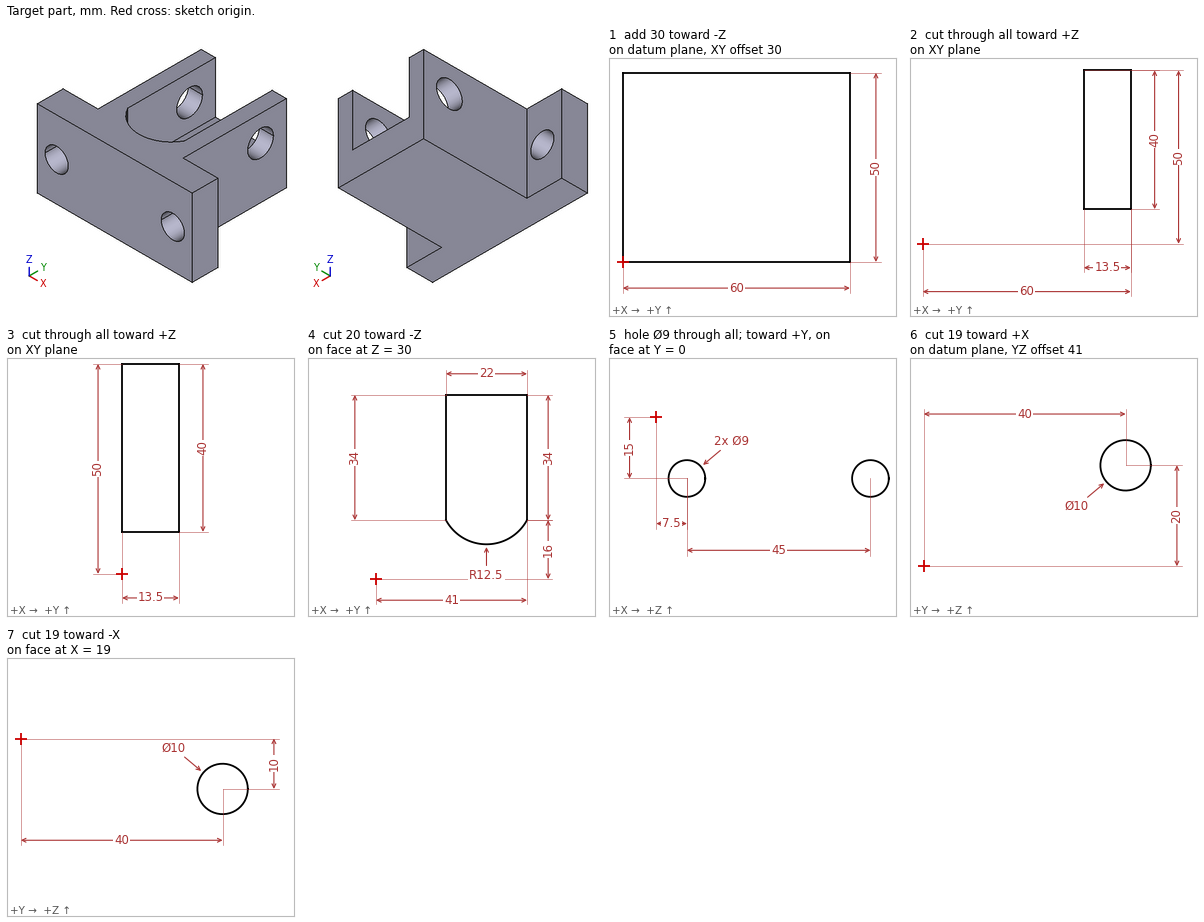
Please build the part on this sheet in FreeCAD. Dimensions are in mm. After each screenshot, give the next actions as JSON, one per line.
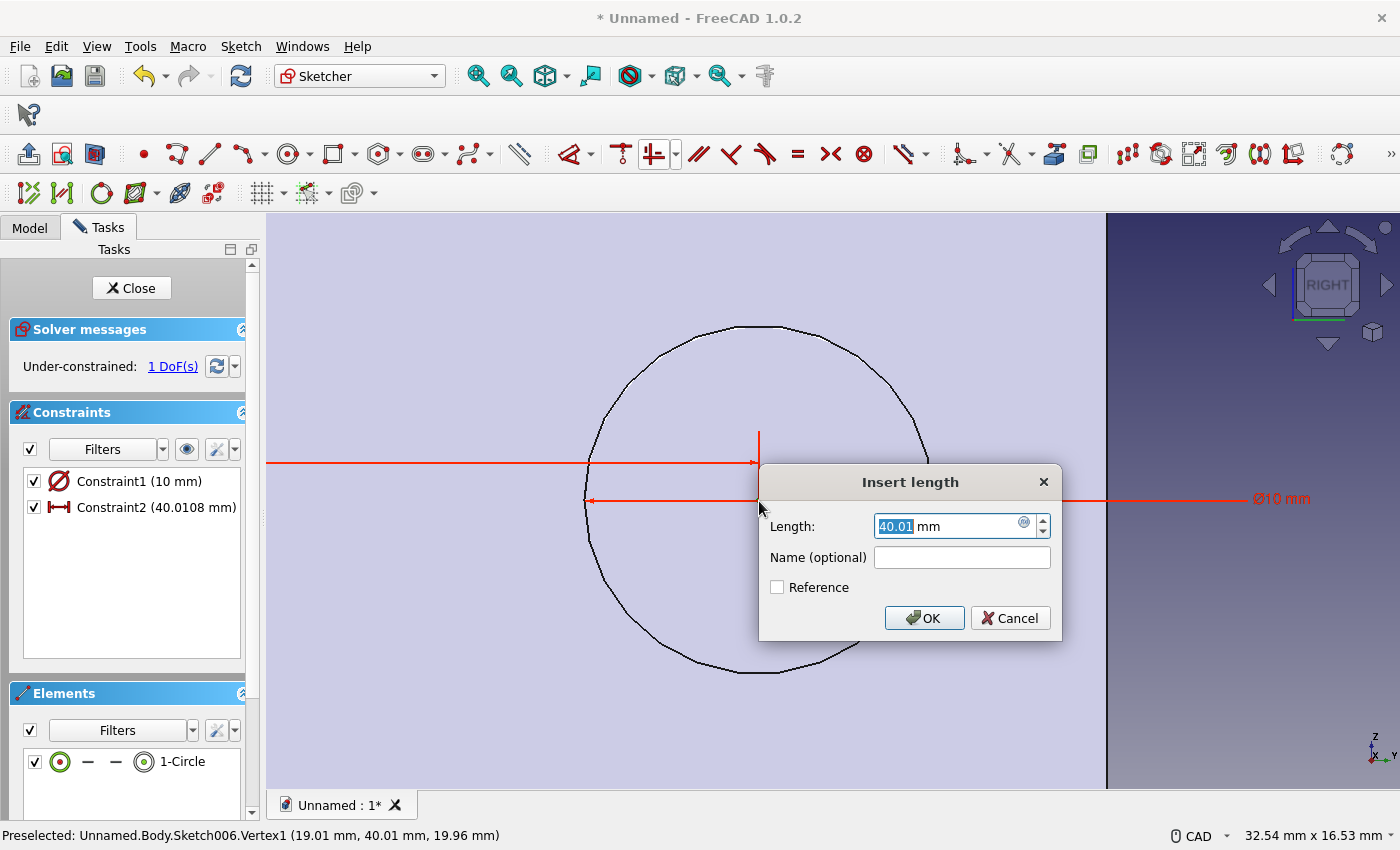
{"action": "type", "text": "40"}
{"action": "key", "text": "Return"}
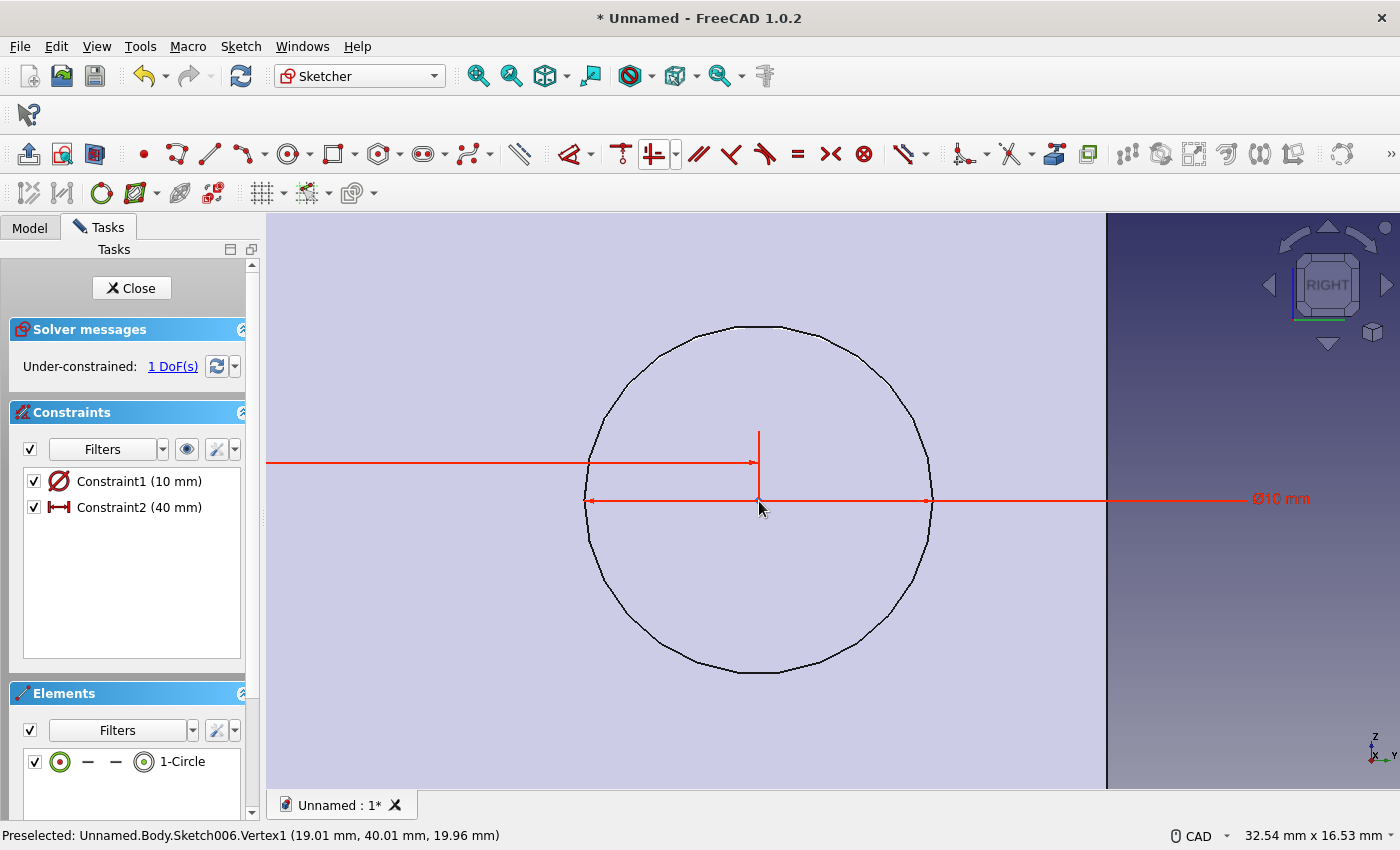
{"action": "left_click", "coordinate": [759, 501]}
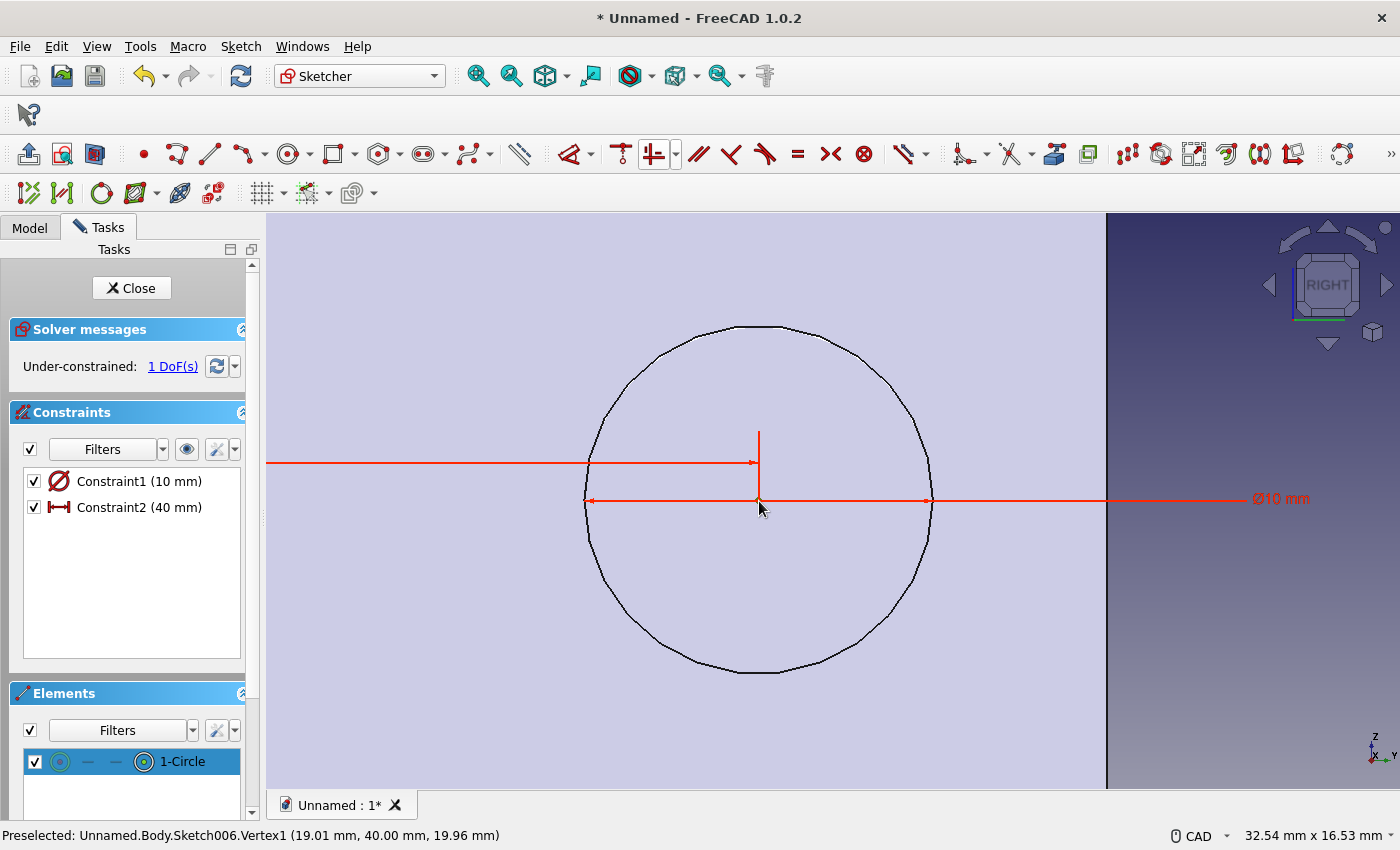
{"action": "key", "text": "i"}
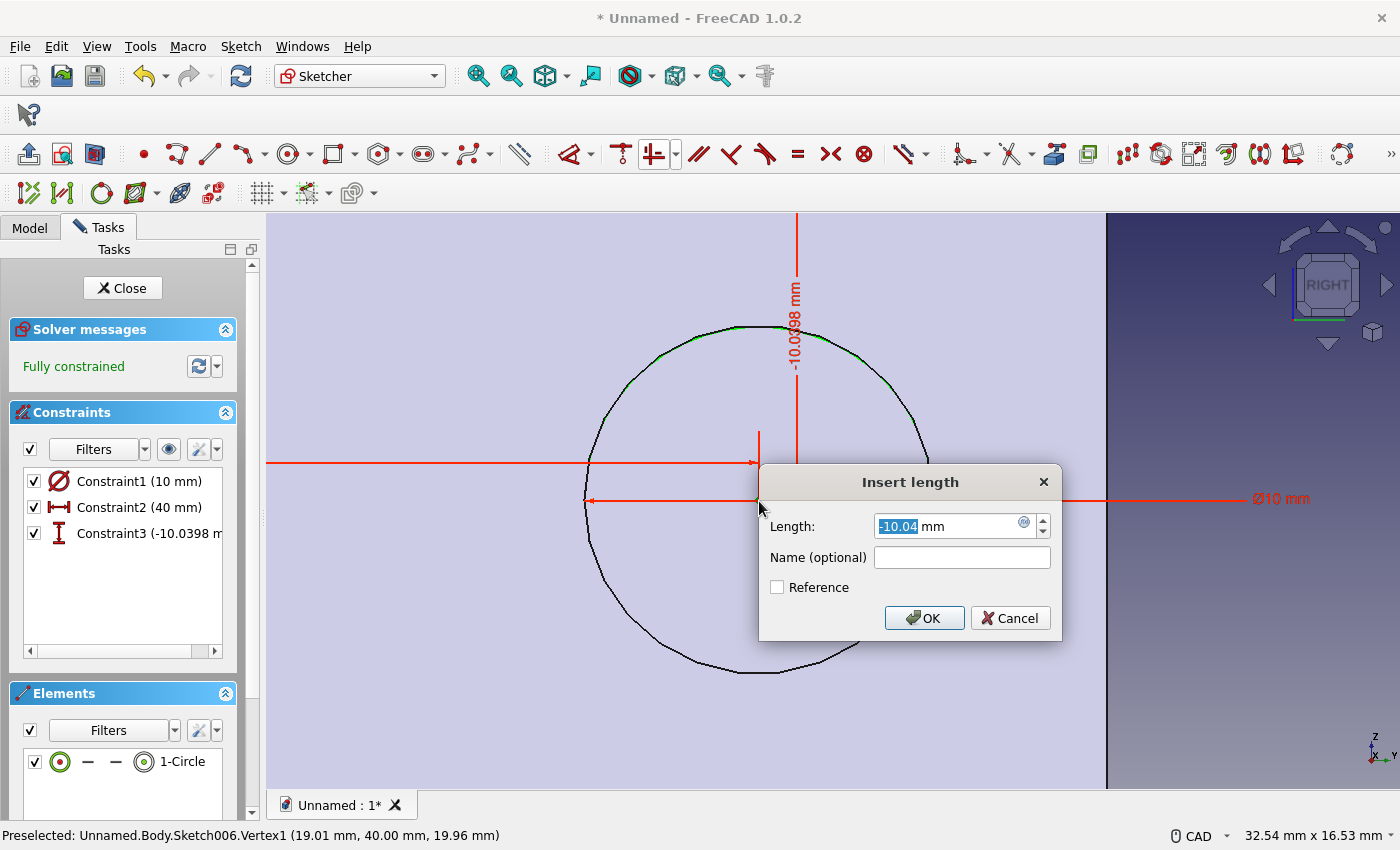
{"action": "type", "text": "-10"}
{"action": "key", "text": "Return"}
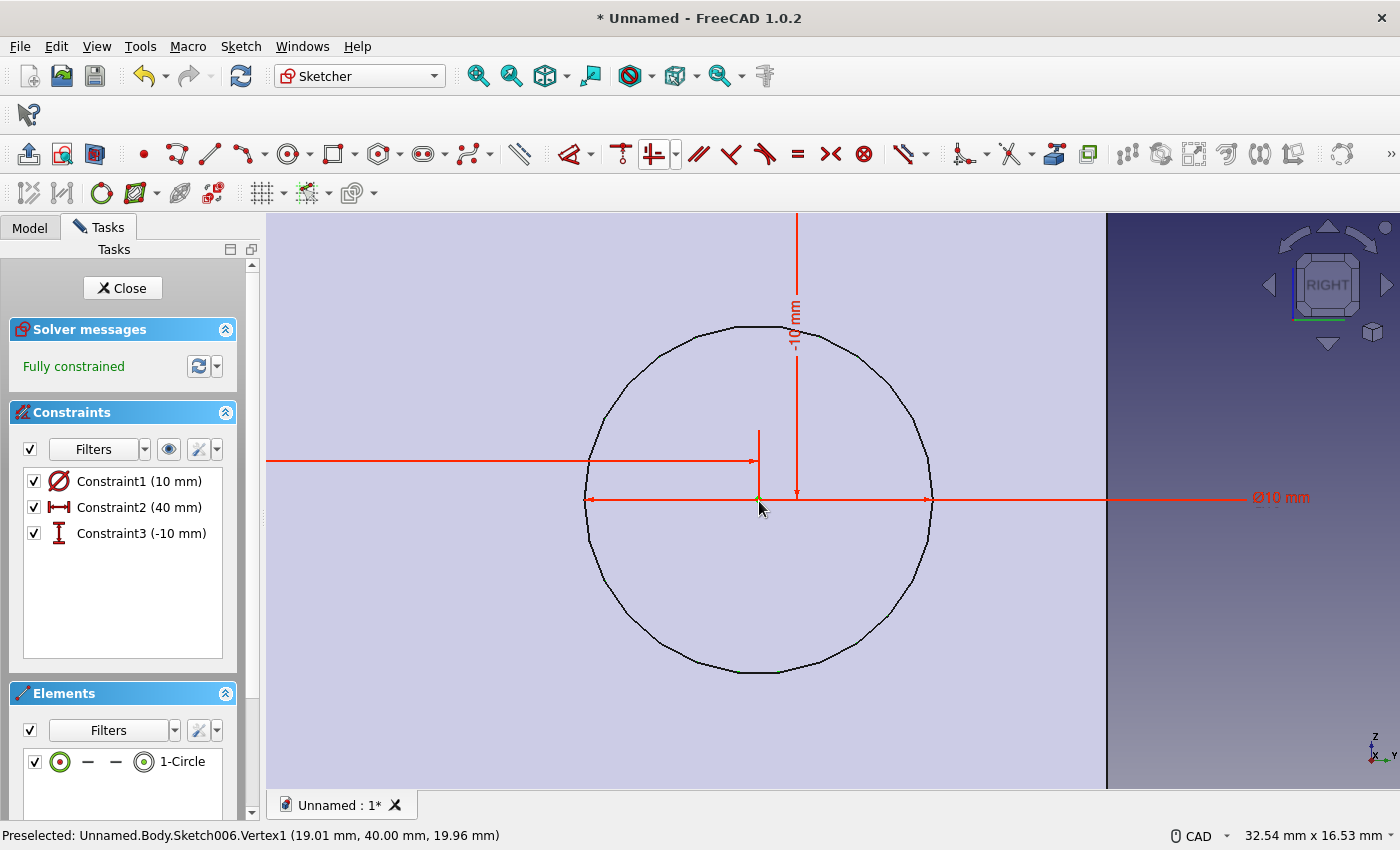
{"action": "left_click", "coordinate": [123, 288]}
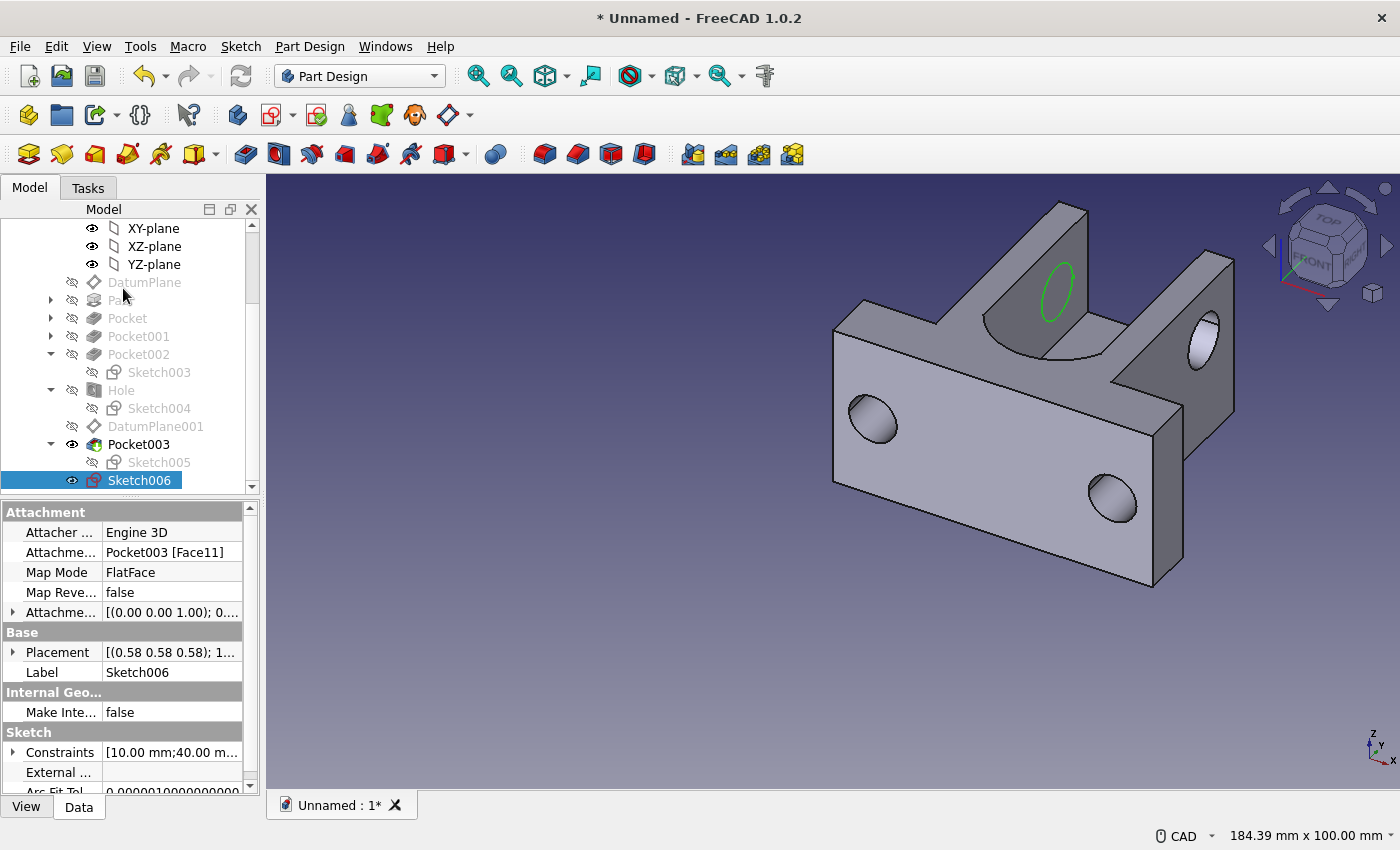
{"action": "left_click", "coordinate": [246, 154]}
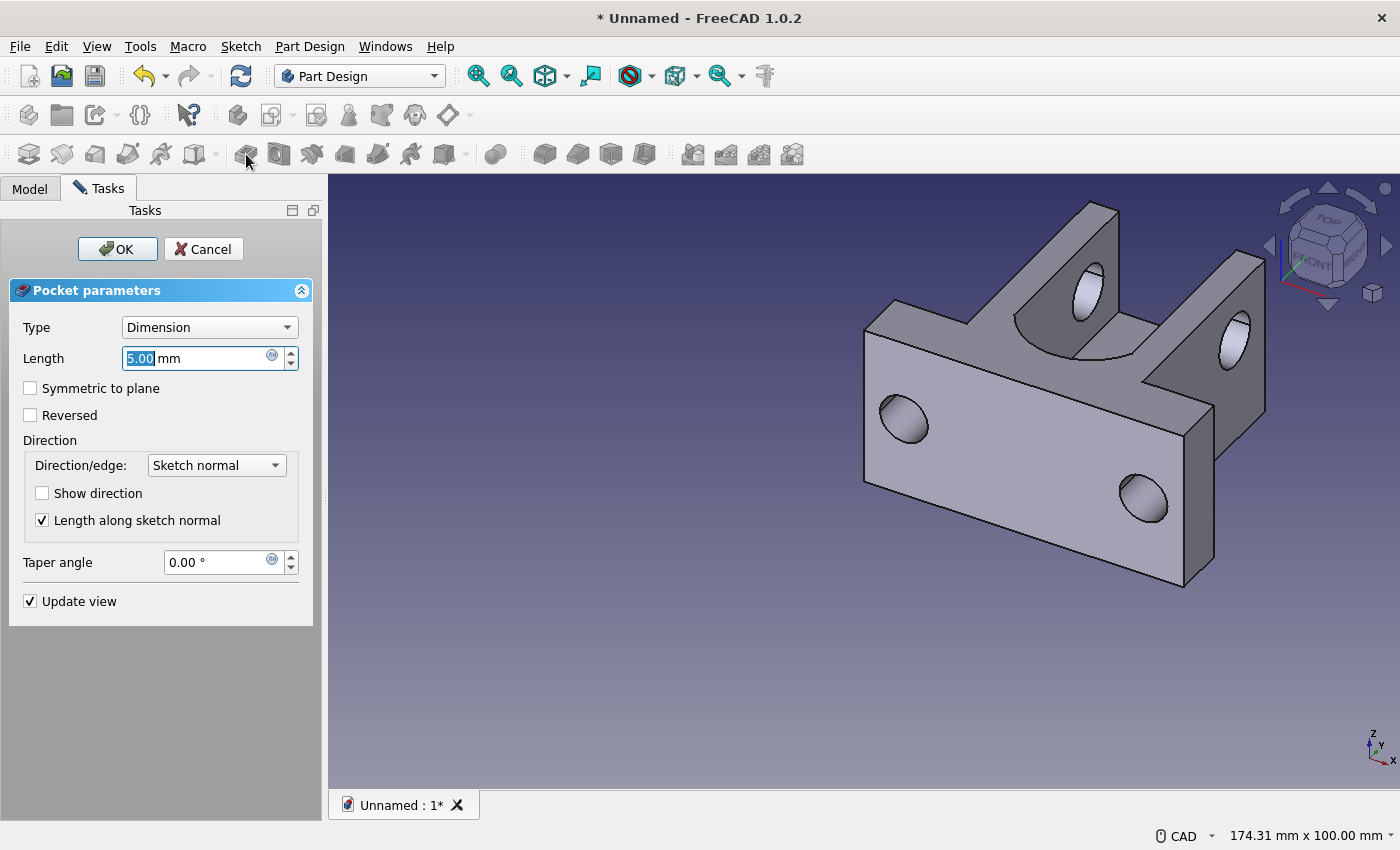
{"action": "type", "text": "19"}
{"action": "key", "text": "Tab"}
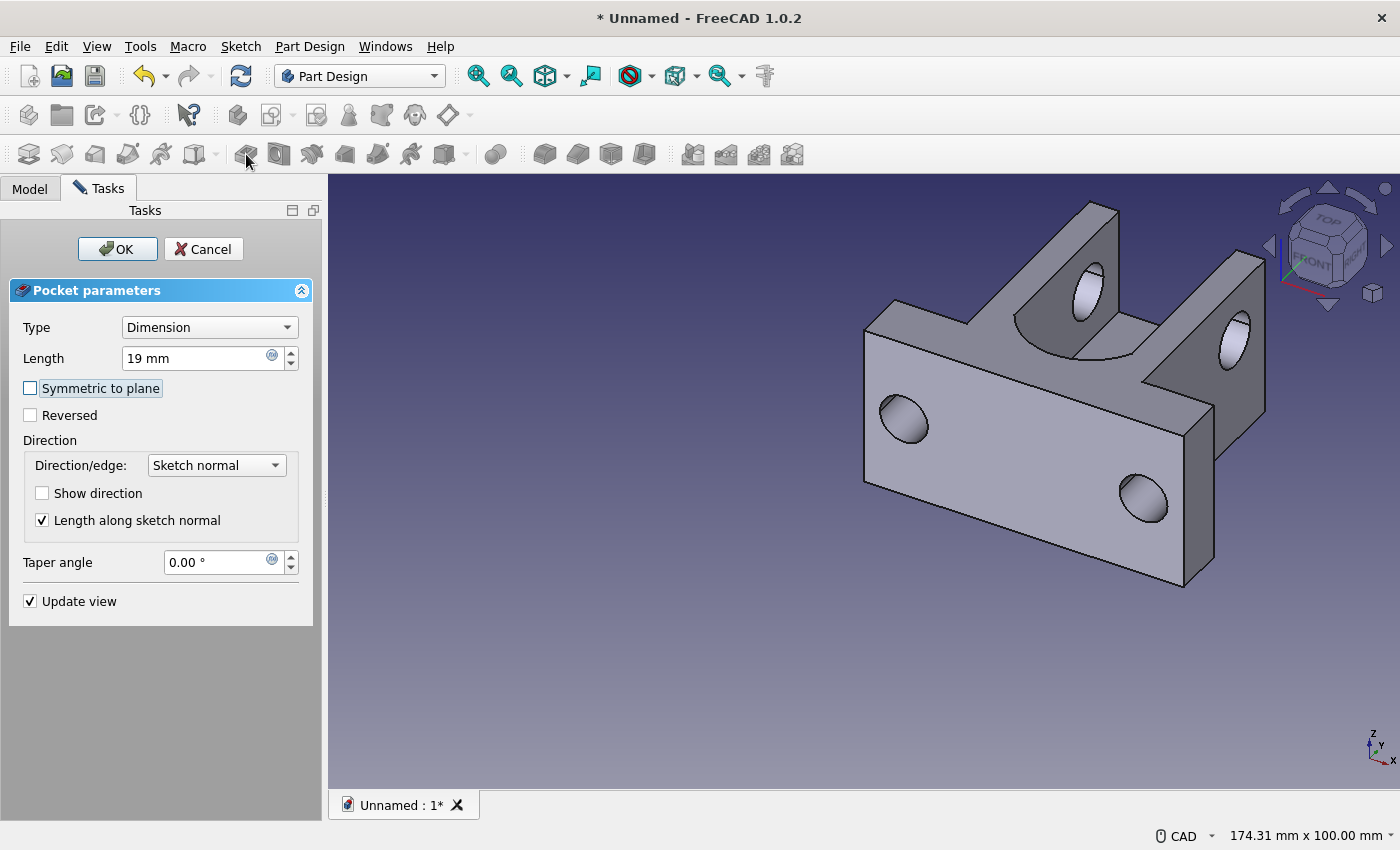
{"action": "left_click", "coordinate": [118, 249]}